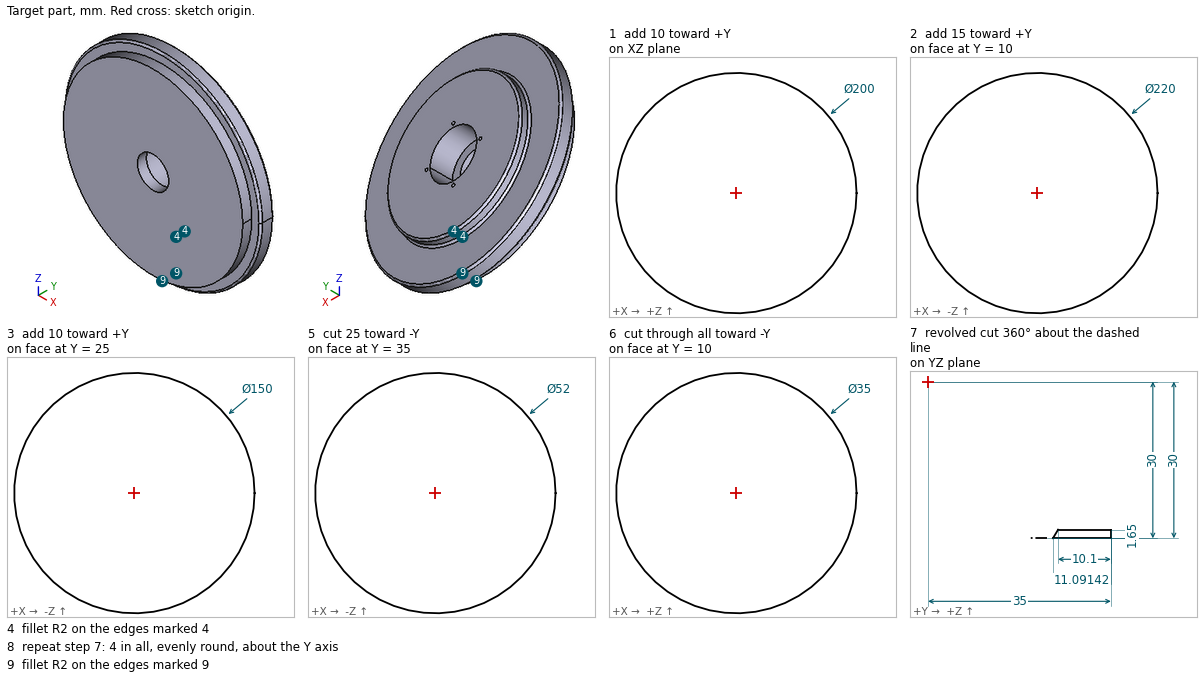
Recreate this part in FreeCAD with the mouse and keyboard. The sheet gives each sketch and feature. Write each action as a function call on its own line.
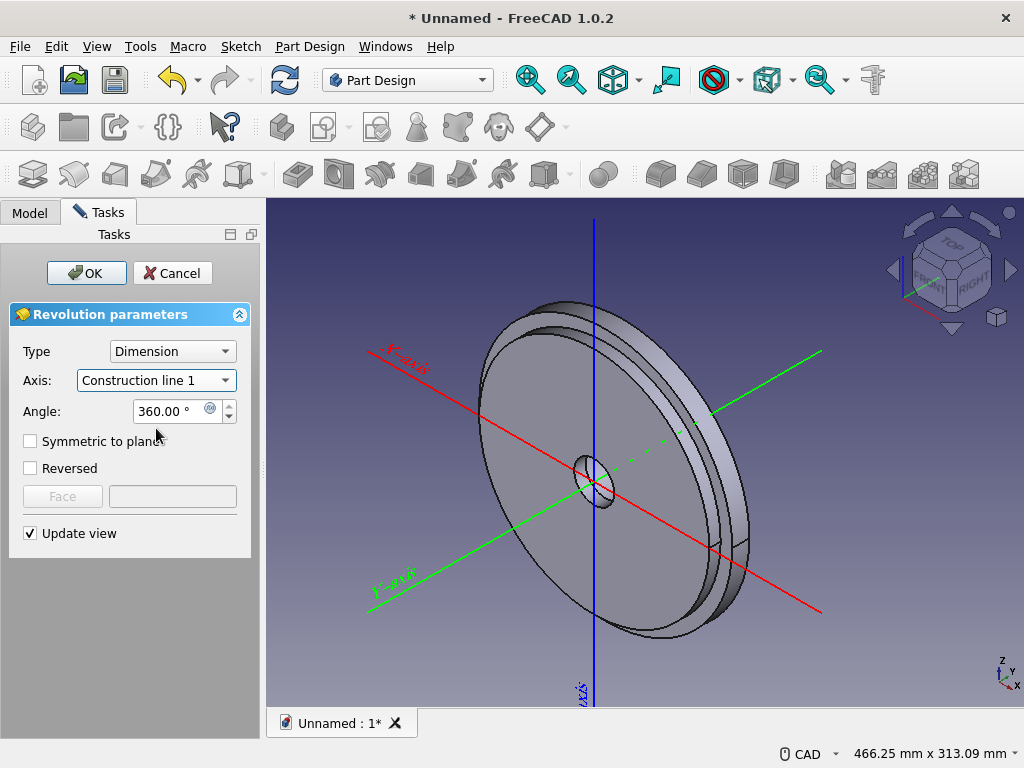
click(87, 273)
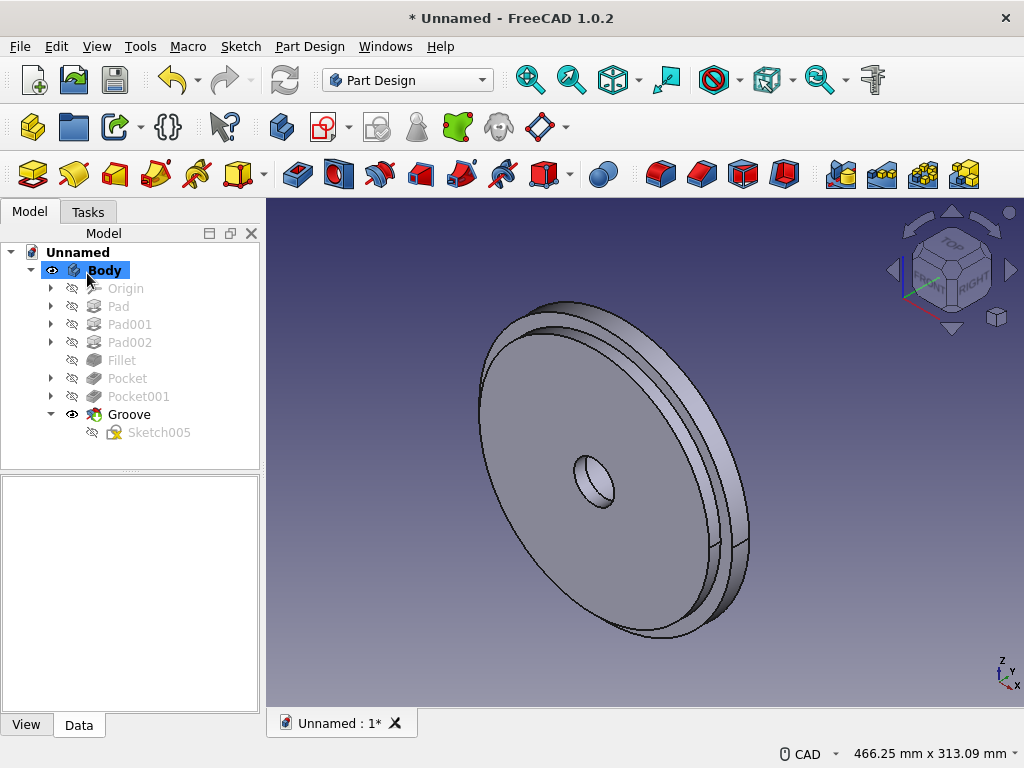
click(117, 414)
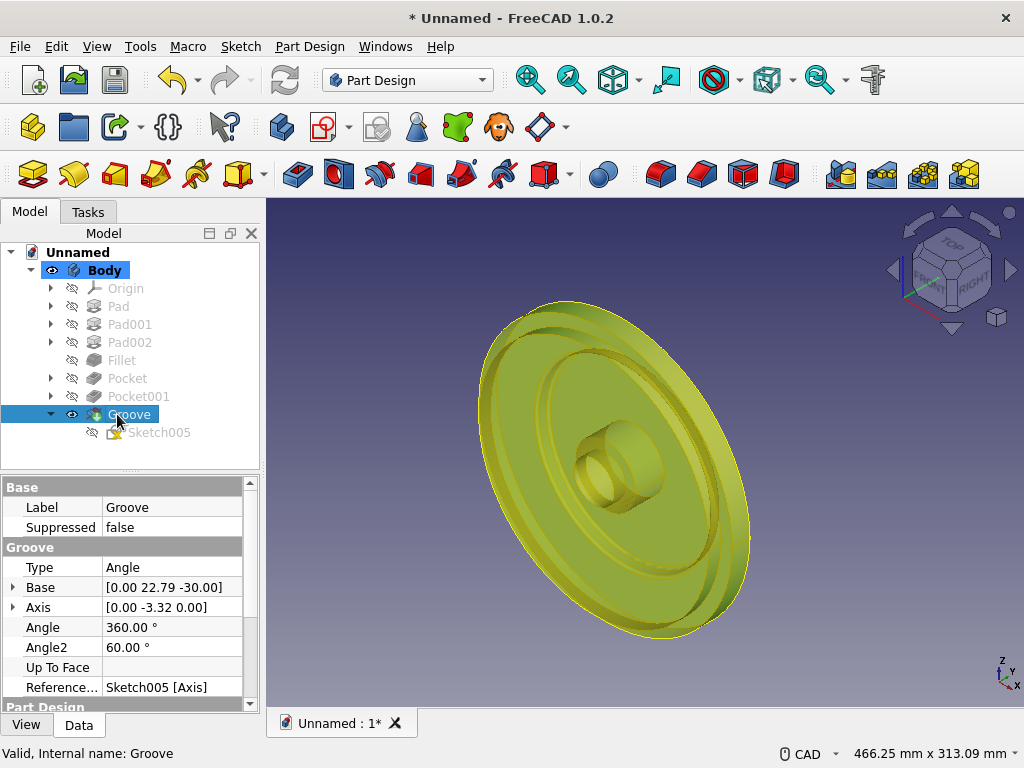
click(923, 174)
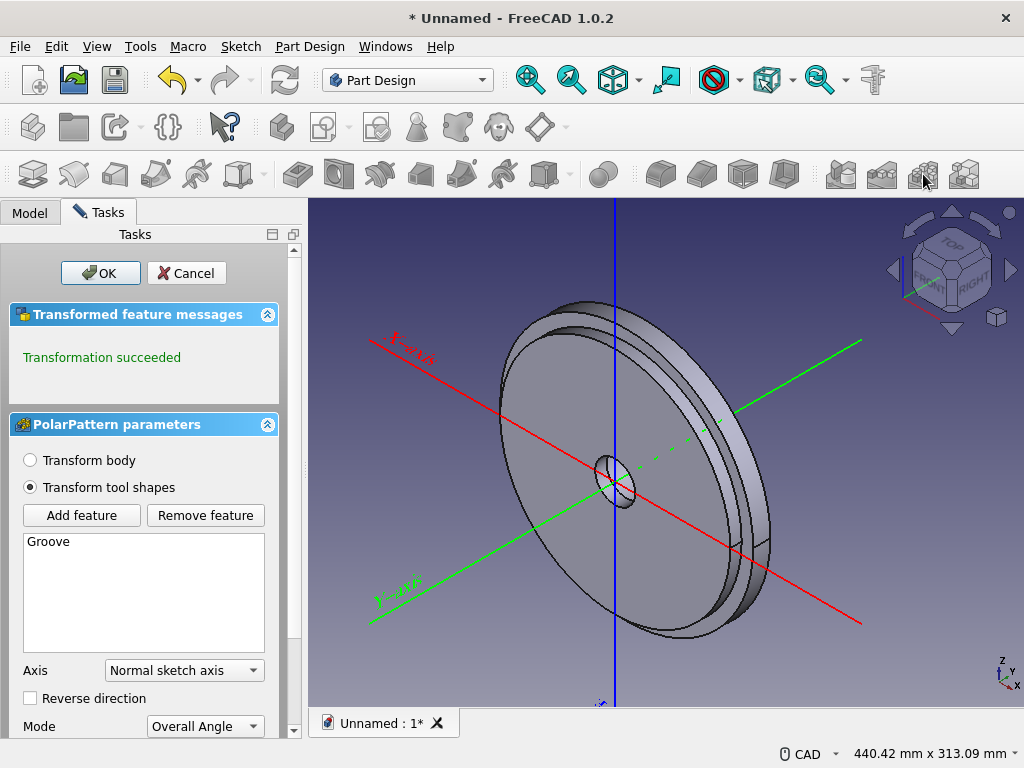
click(185, 670)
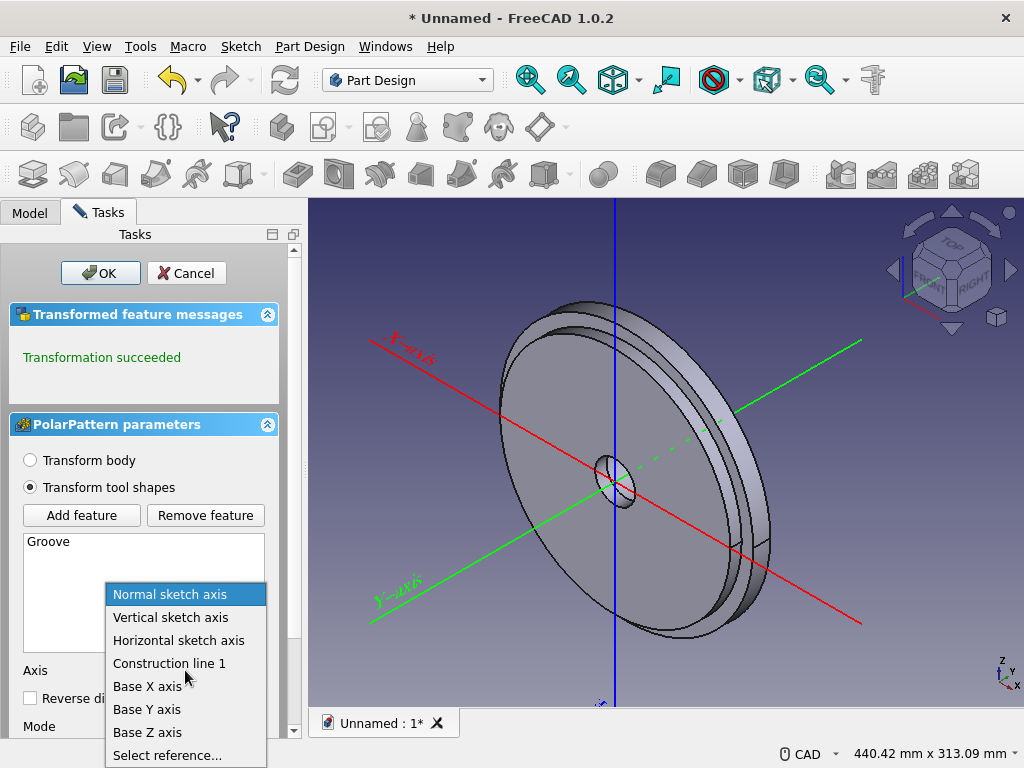
click(184, 710)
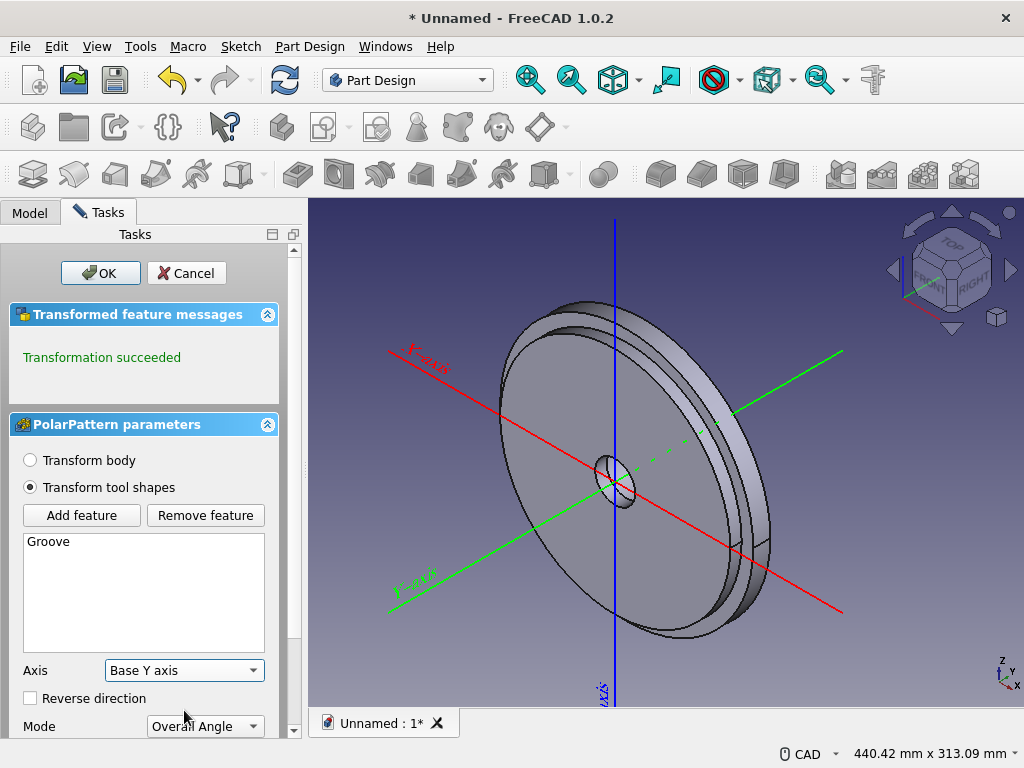
scroll(294, 491, down, 3)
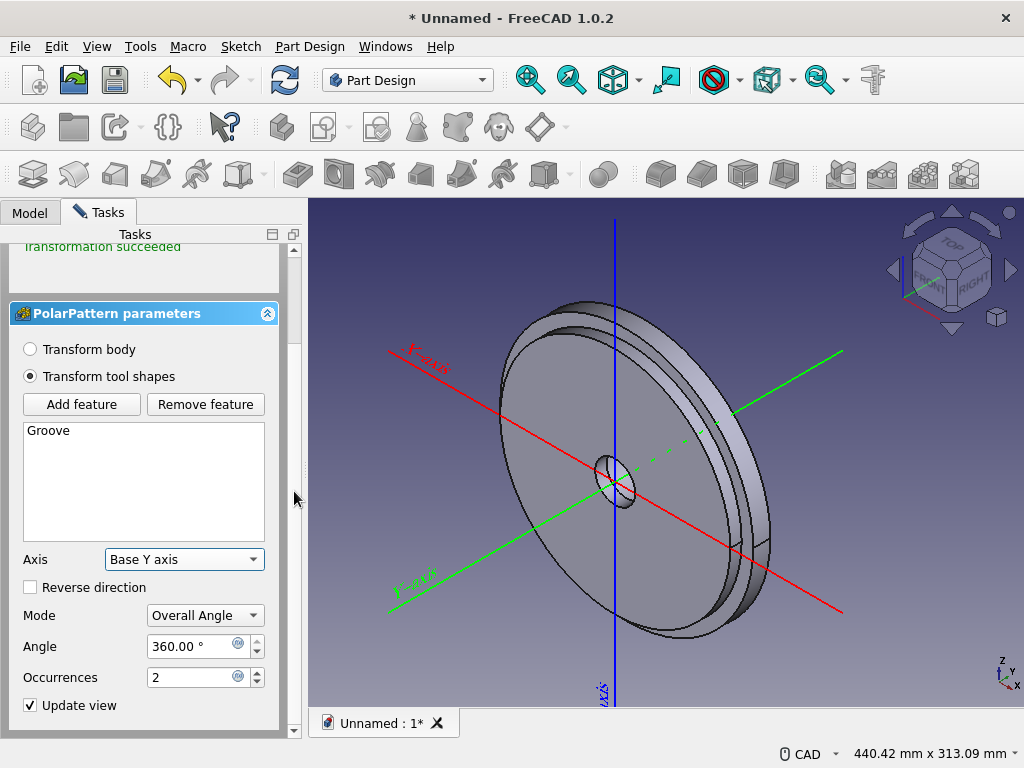
triple_click(199, 678)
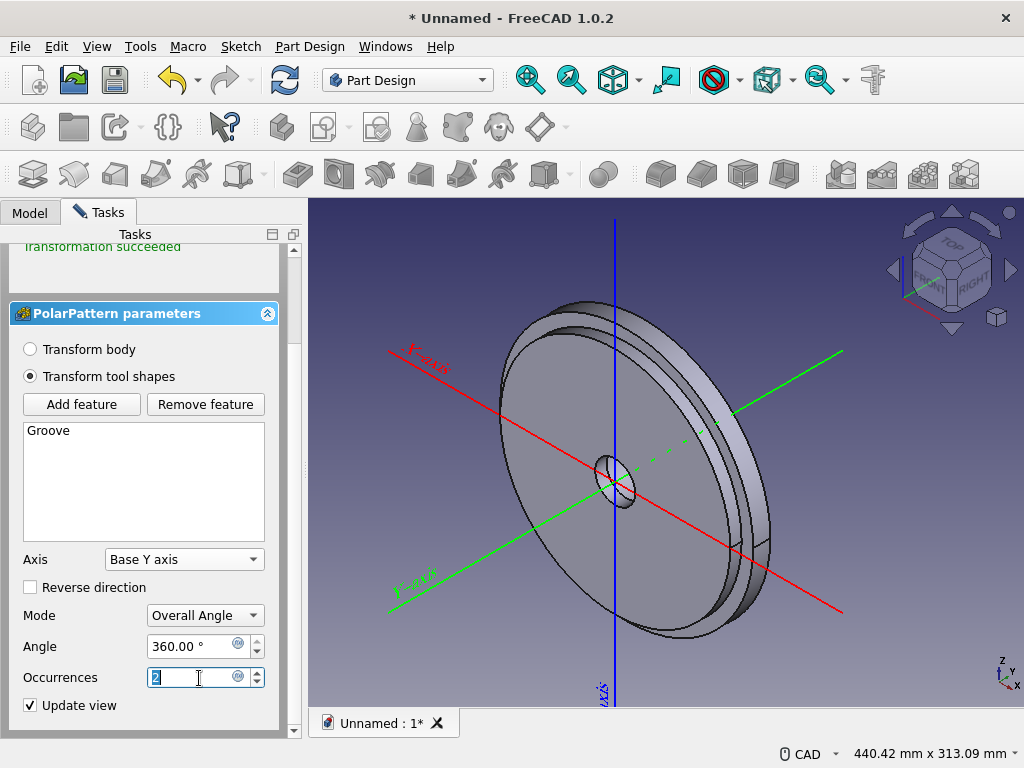
text(4)
key(Tab)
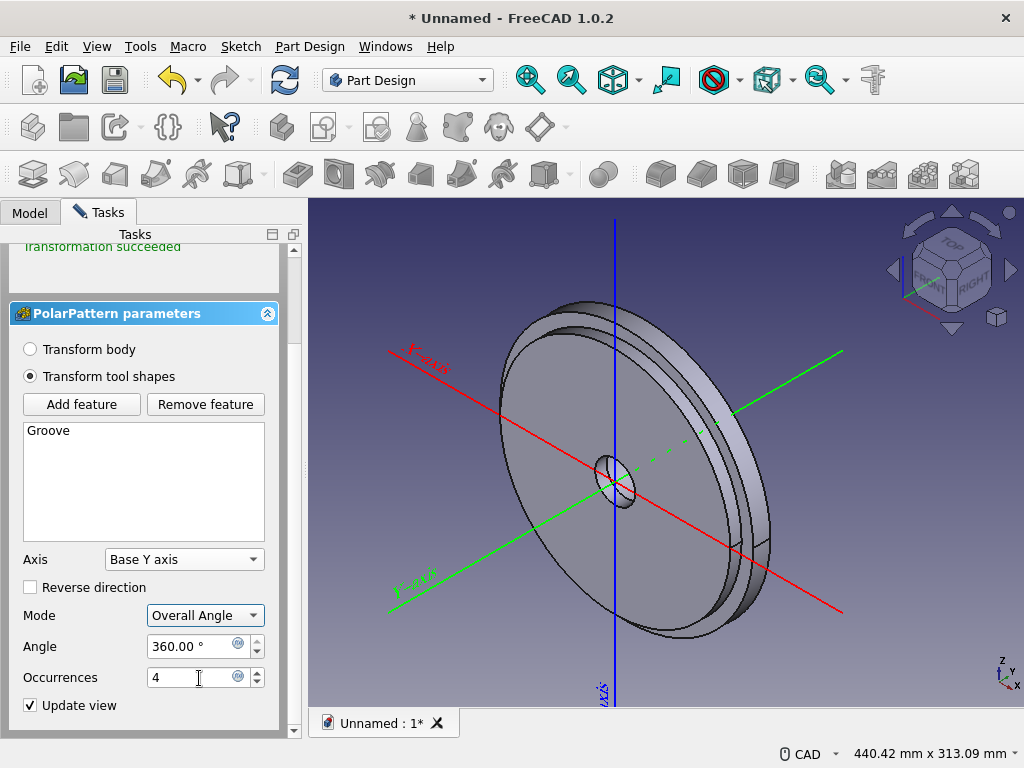
scroll(294, 491, up, 3)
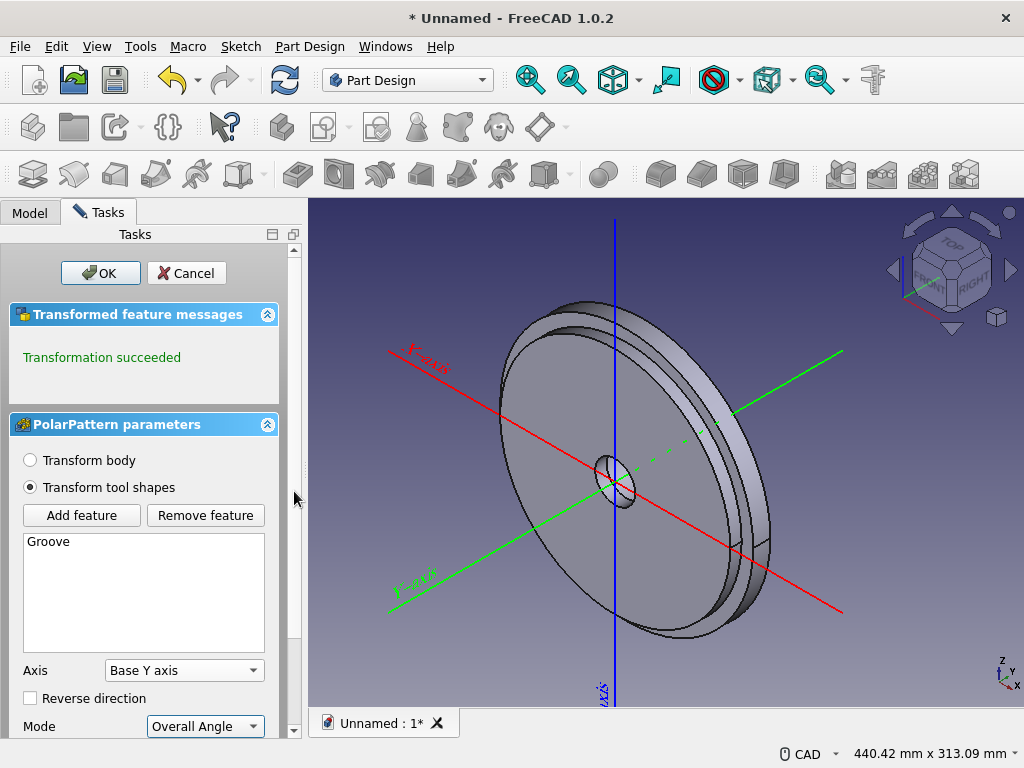
click(101, 273)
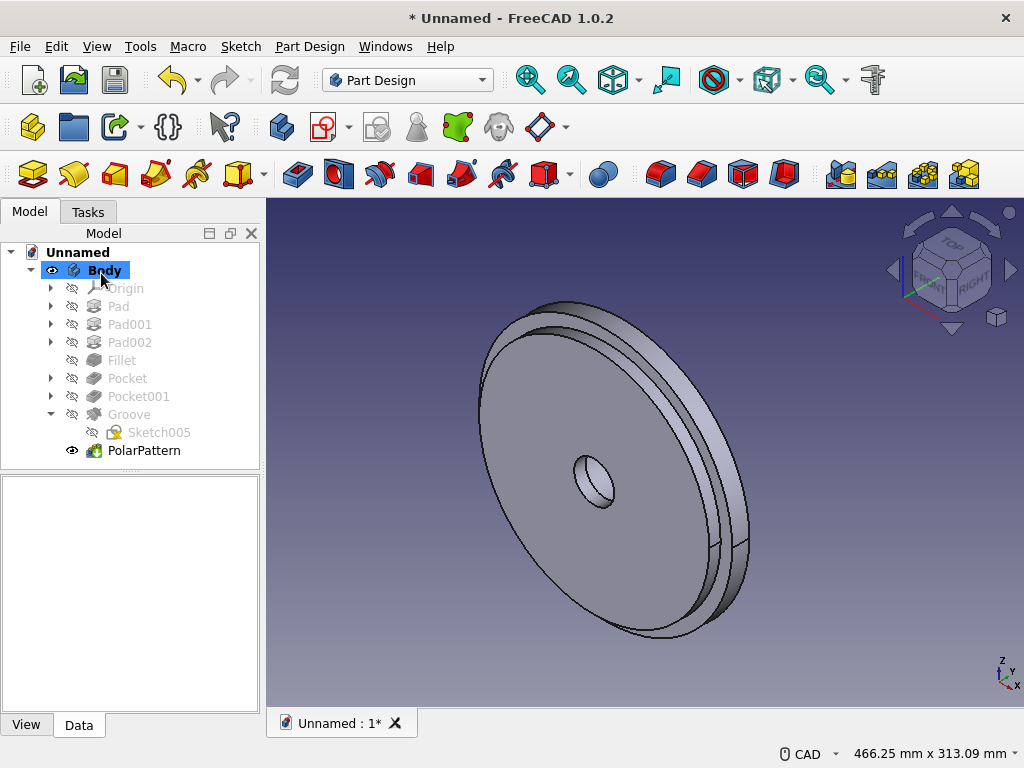
click(567, 313)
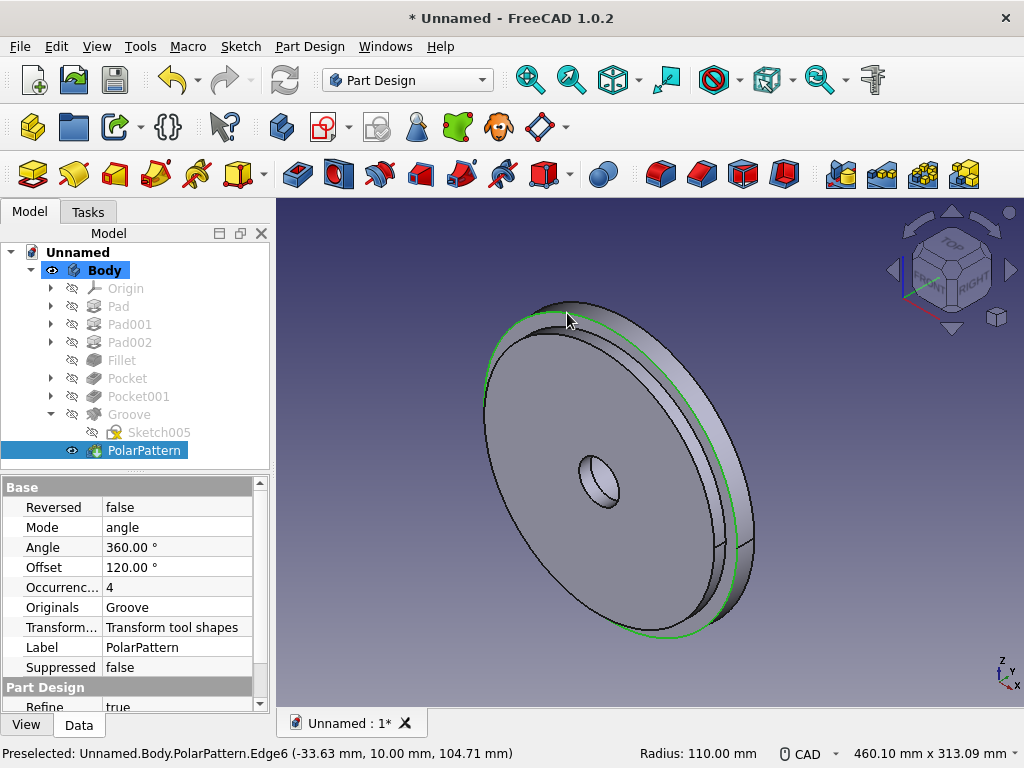
key(2)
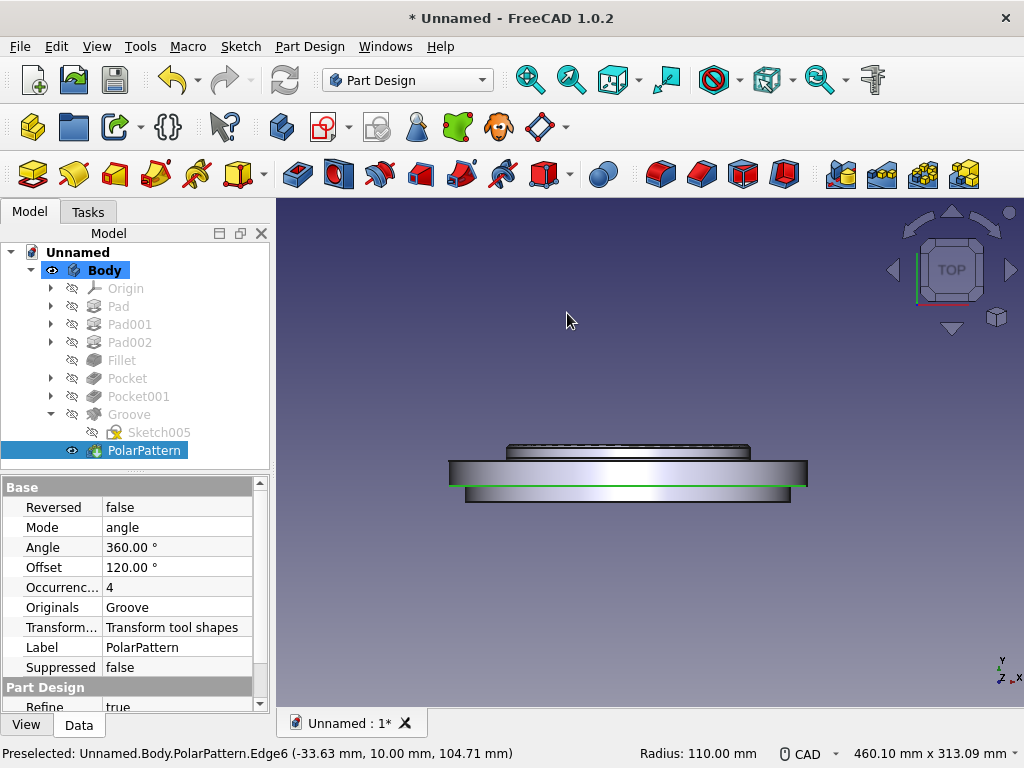
click(483, 460, ctrl)